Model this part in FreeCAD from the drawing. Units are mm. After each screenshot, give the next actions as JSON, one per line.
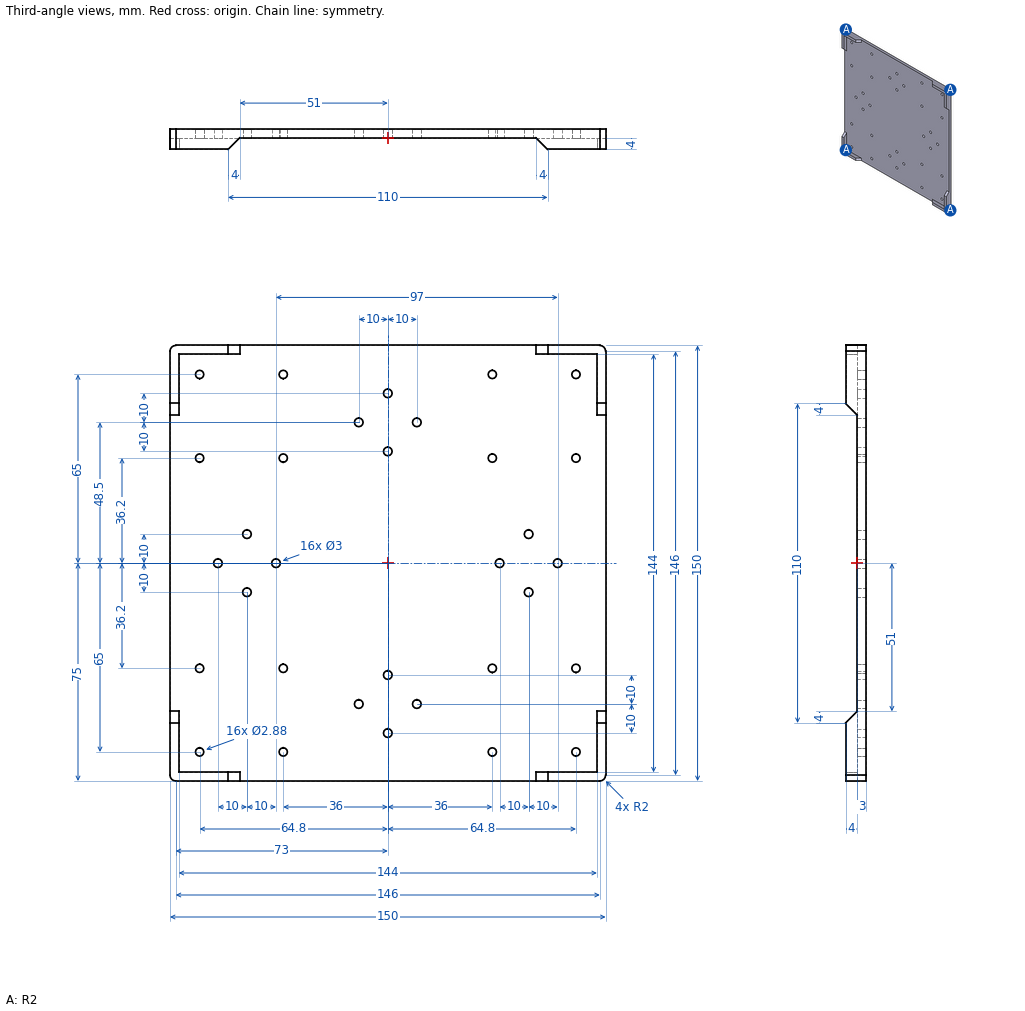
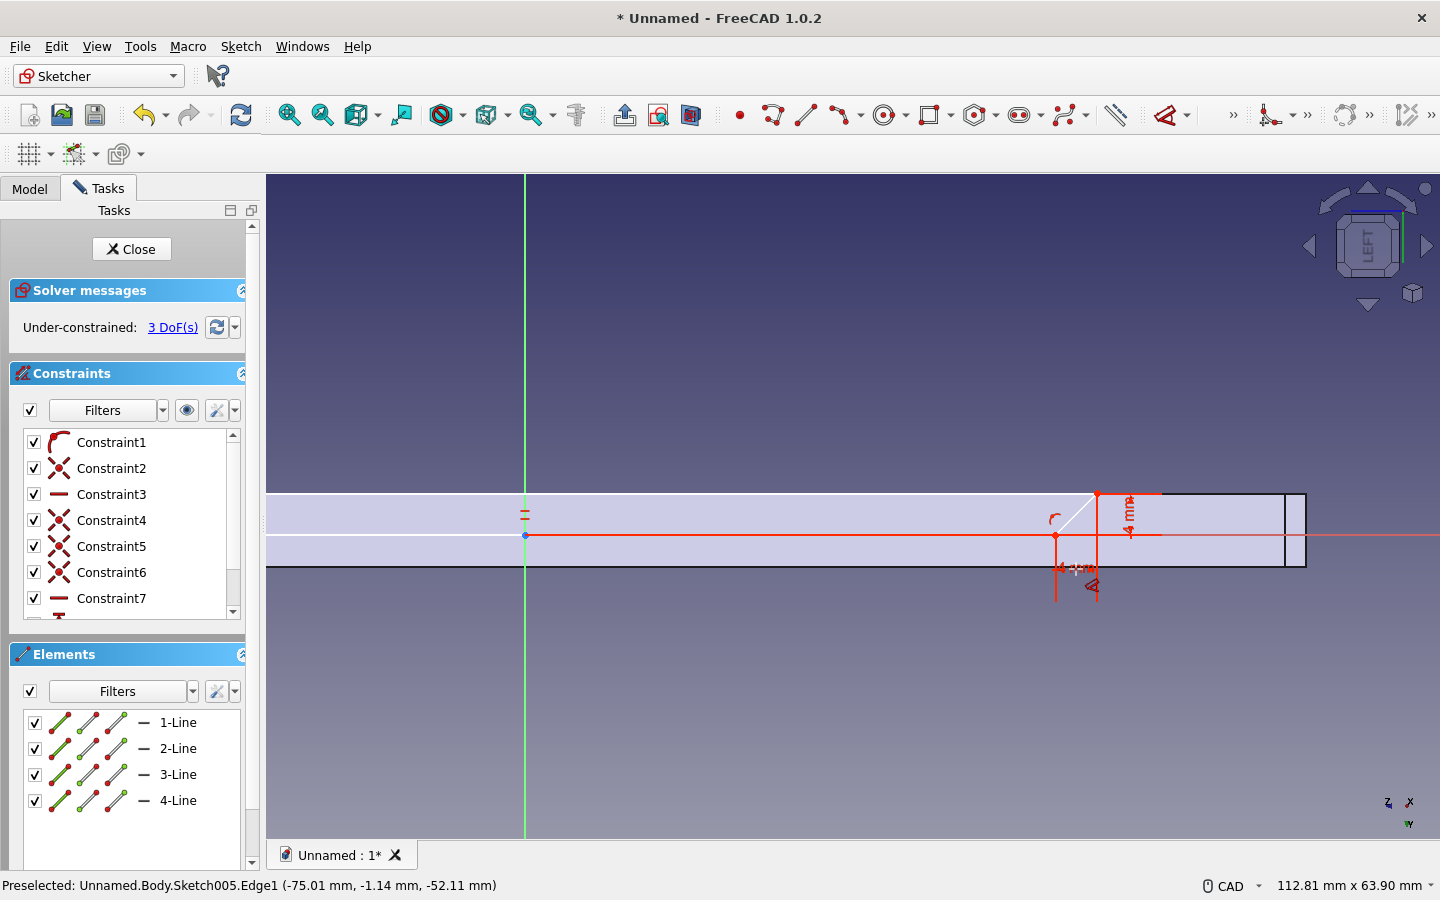
{"action": "scroll", "coordinate": [1100, 497], "scroll_direction": "down", "scroll_amount": 3}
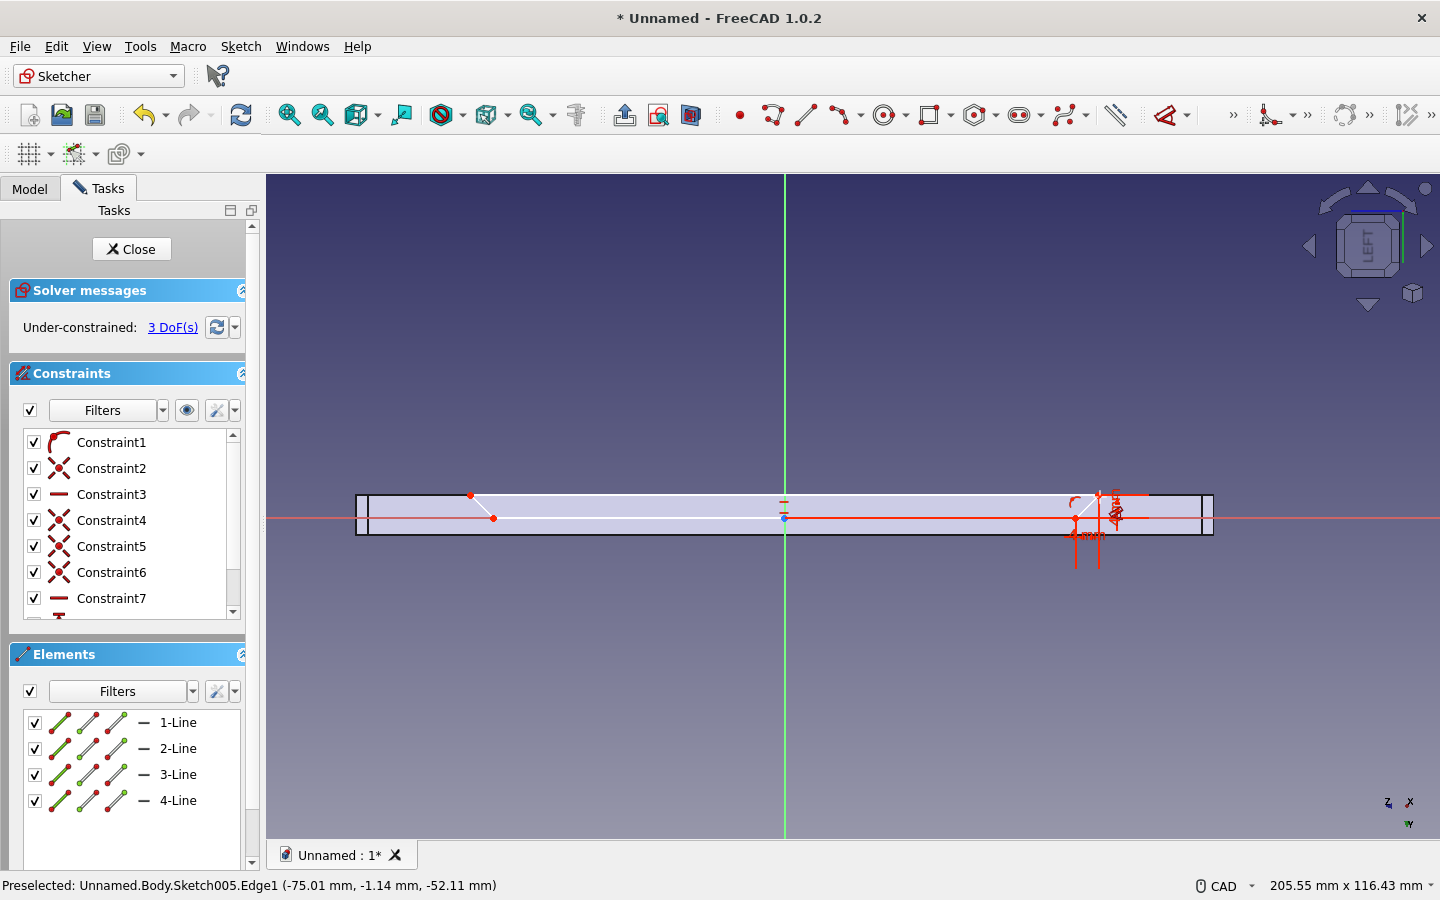
{"action": "scroll", "coordinate": [478, 502], "scroll_direction": "up", "scroll_amount": 4}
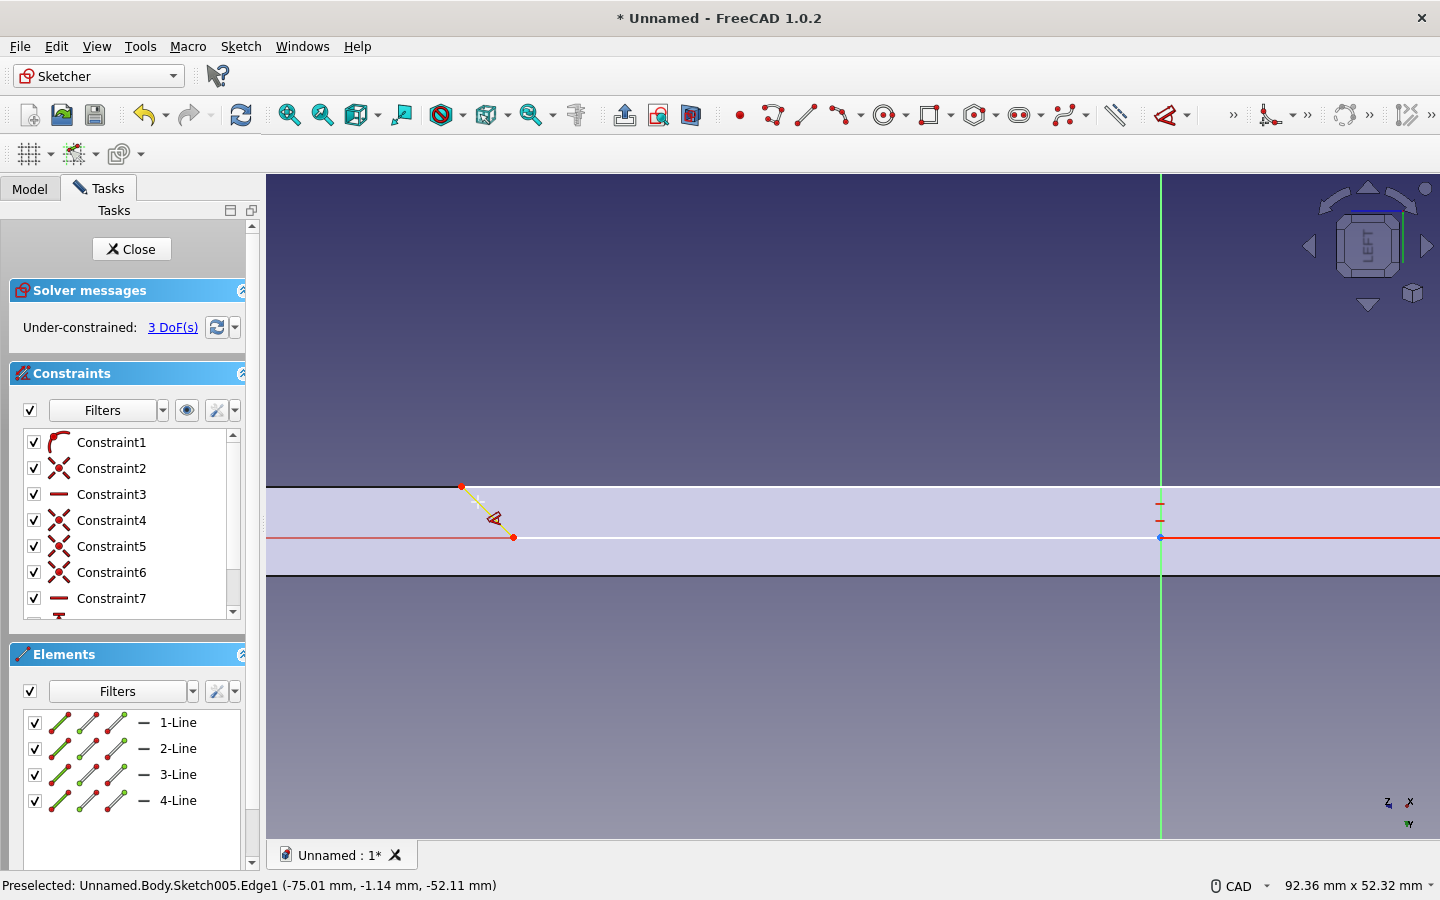
{"action": "left_click", "coordinate": [477, 502]}
{"action": "left_click", "coordinate": [488, 572]}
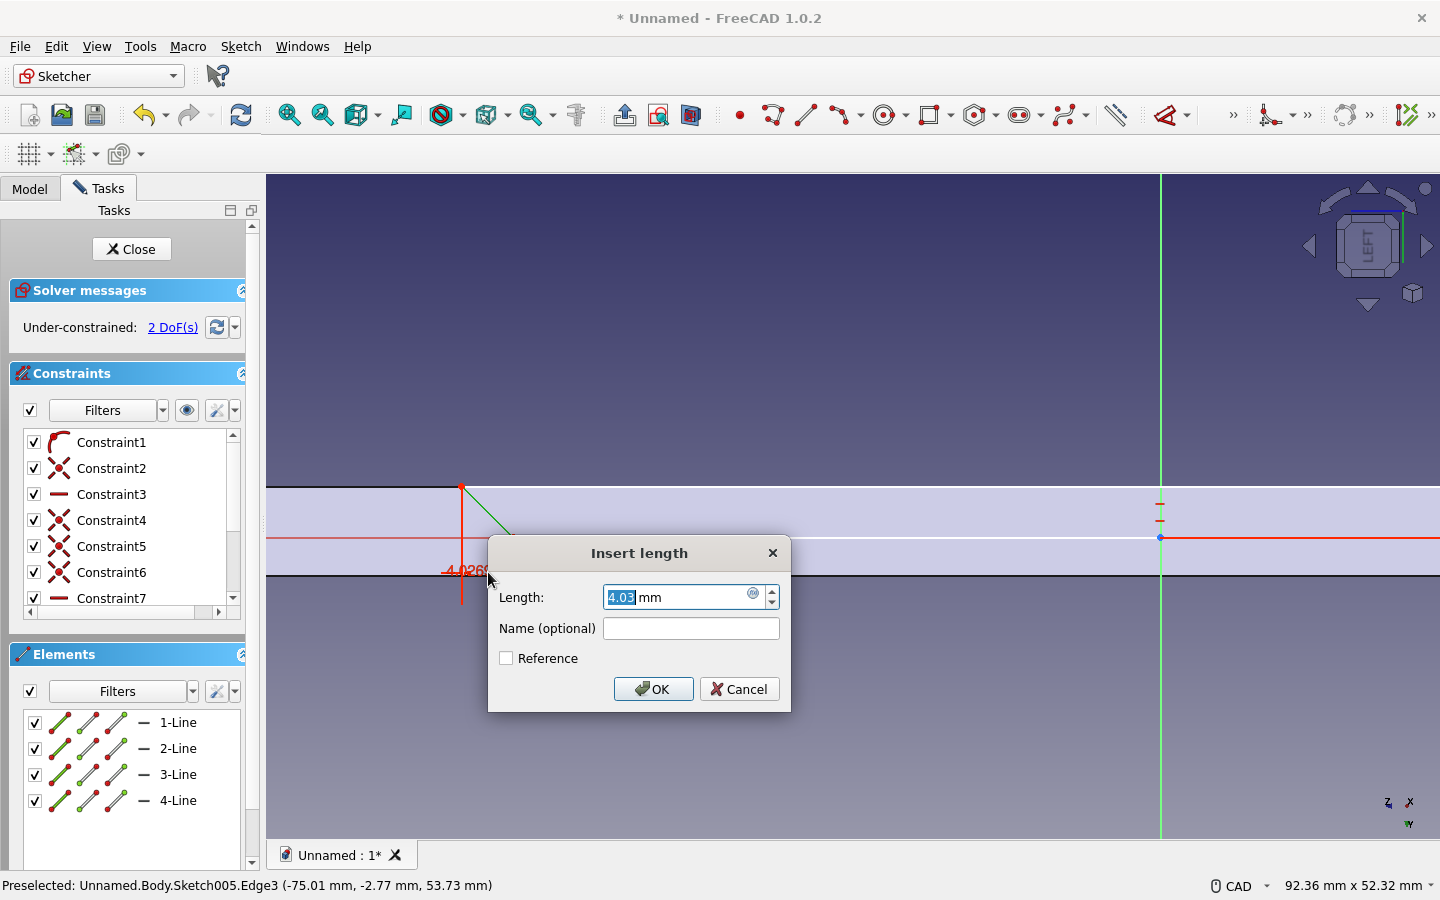
{"action": "type", "text": "4"}
{"action": "key", "text": "Return"}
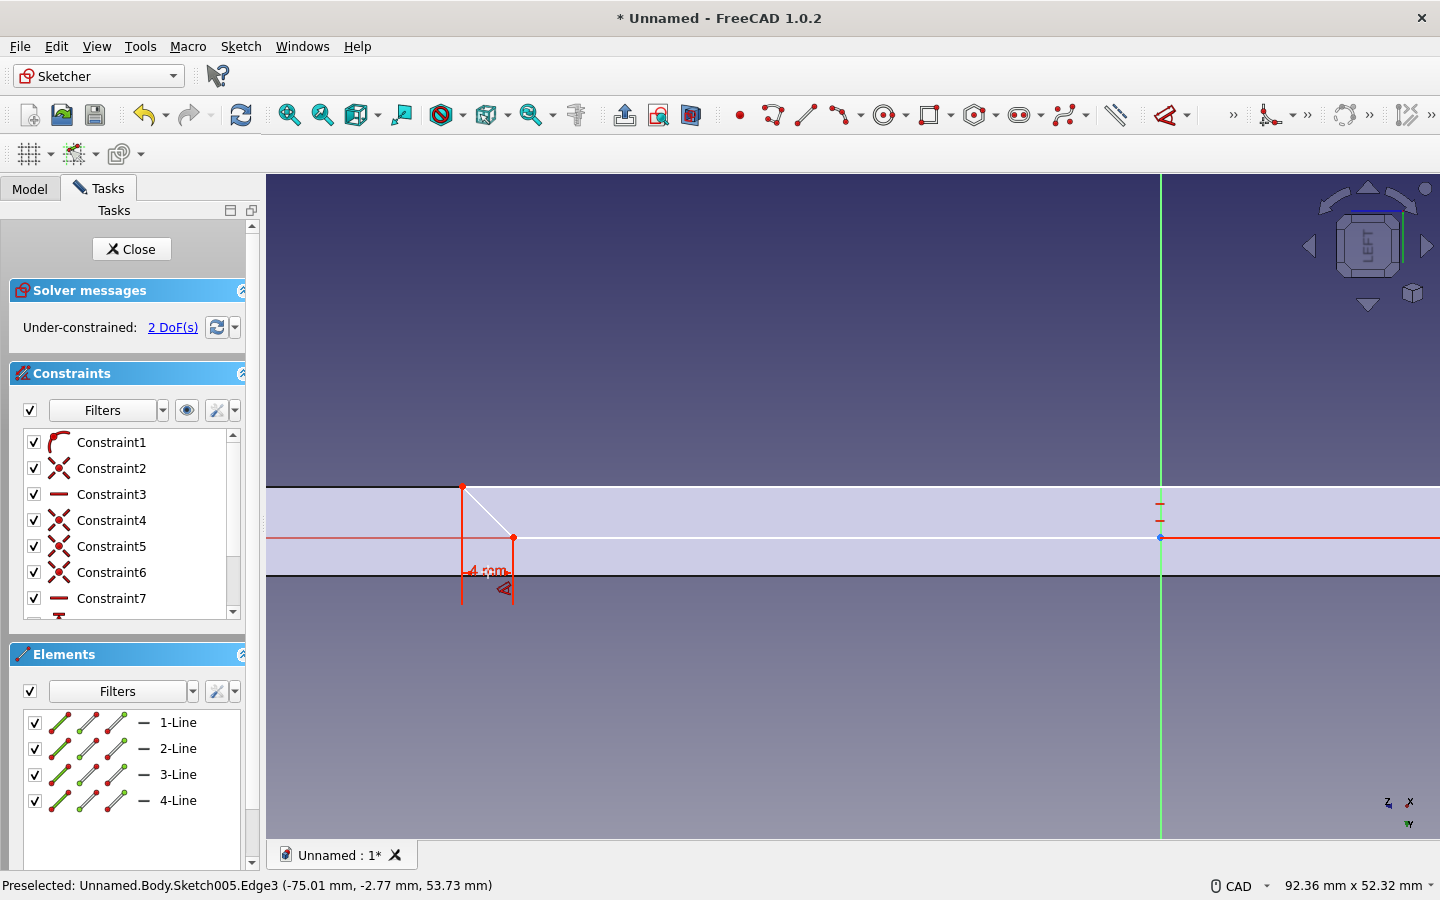
{"action": "left_click", "coordinate": [881, 487]}
{"action": "left_click", "coordinate": [869, 453]}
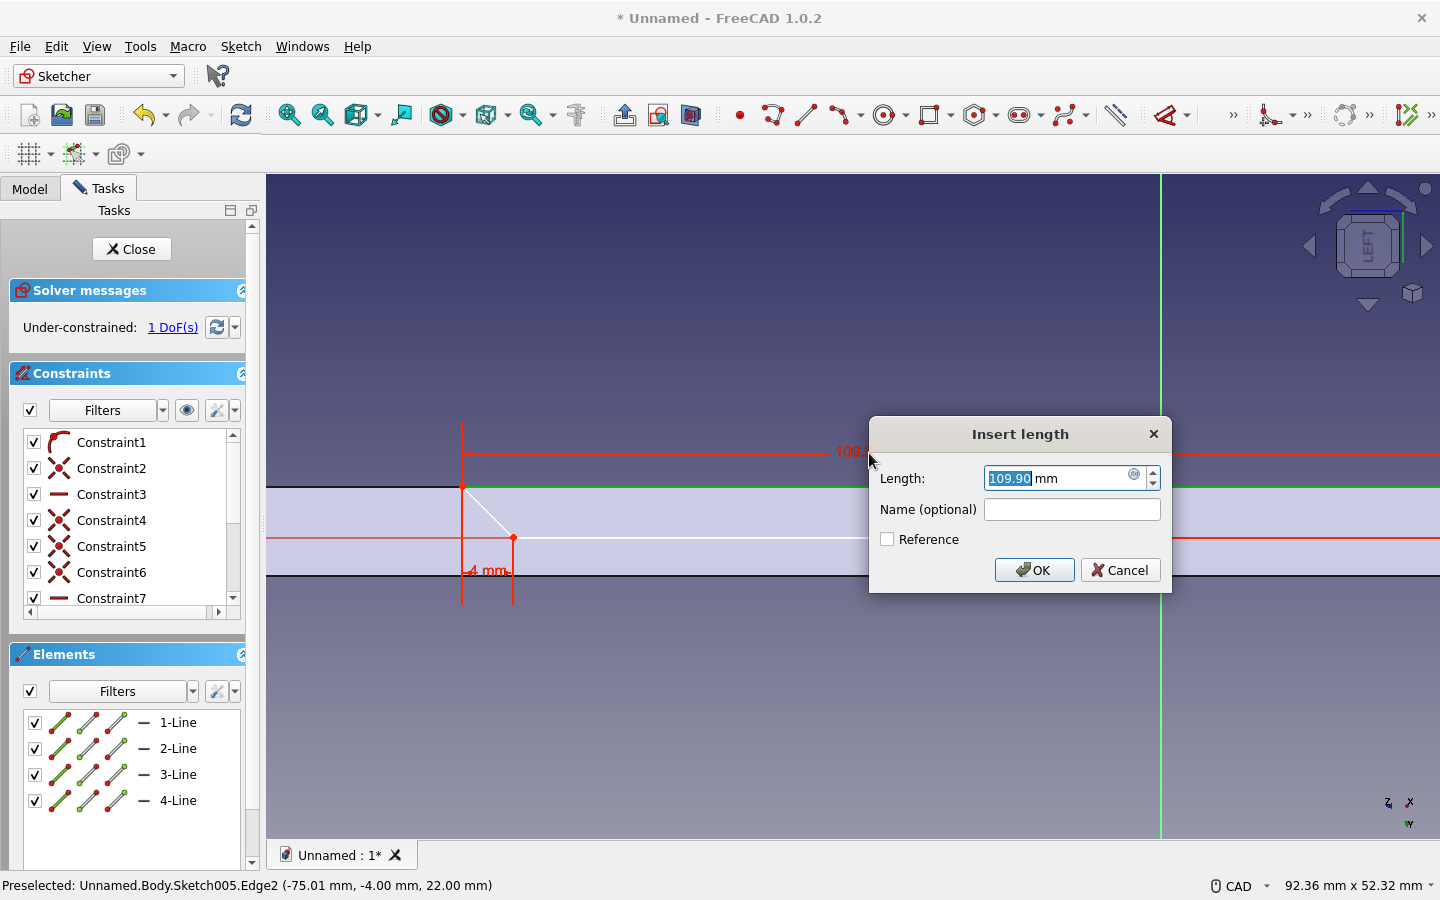
{"action": "type", "text": "110"}
{"action": "key", "text": "Return"}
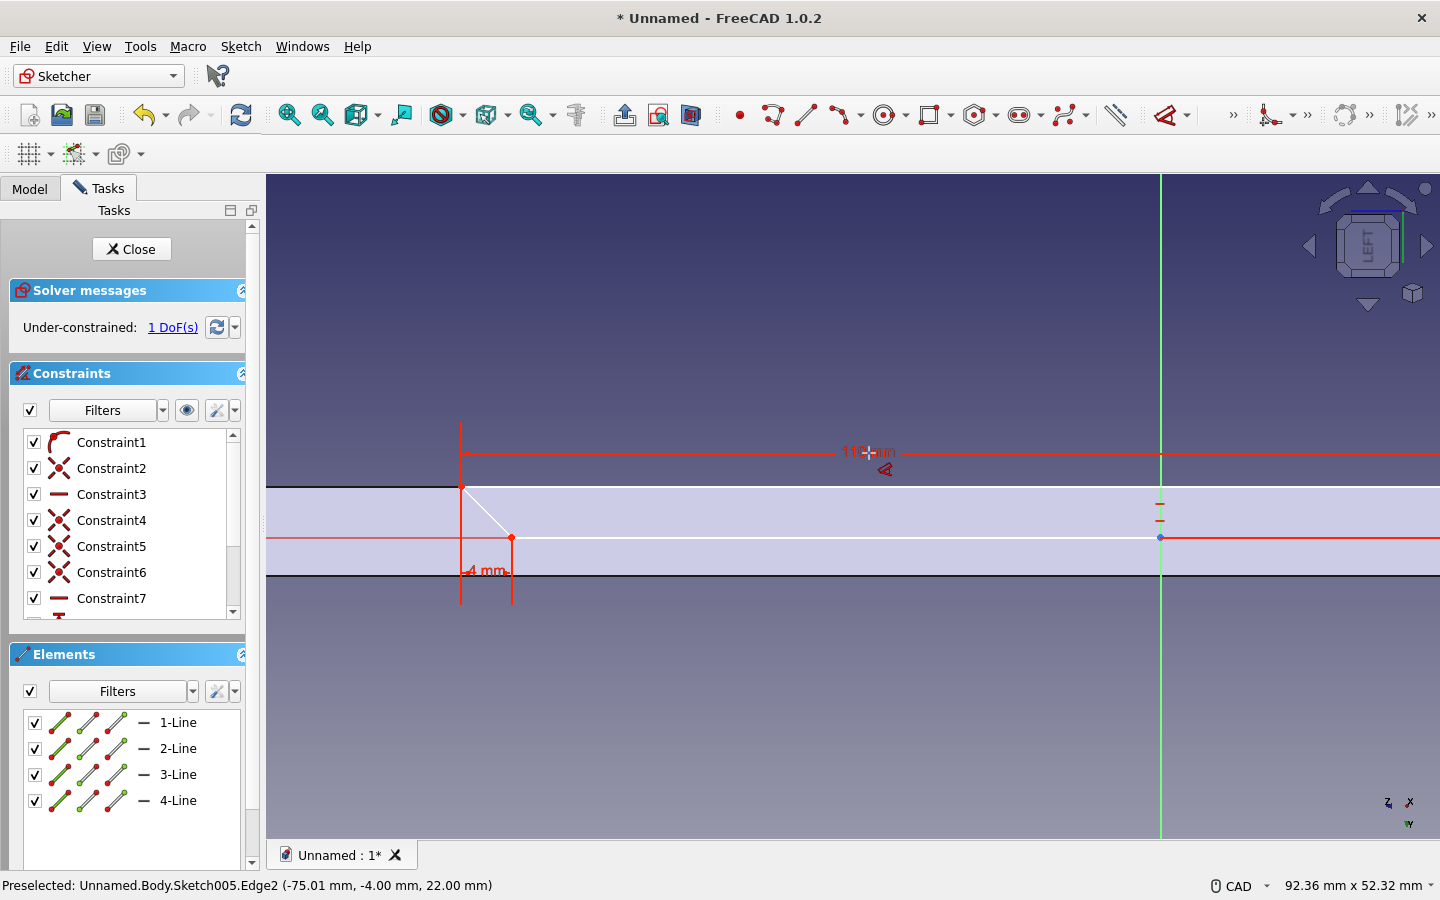
{"action": "scroll", "coordinate": [478, 502], "scroll_direction": "down", "scroll_amount": 4}